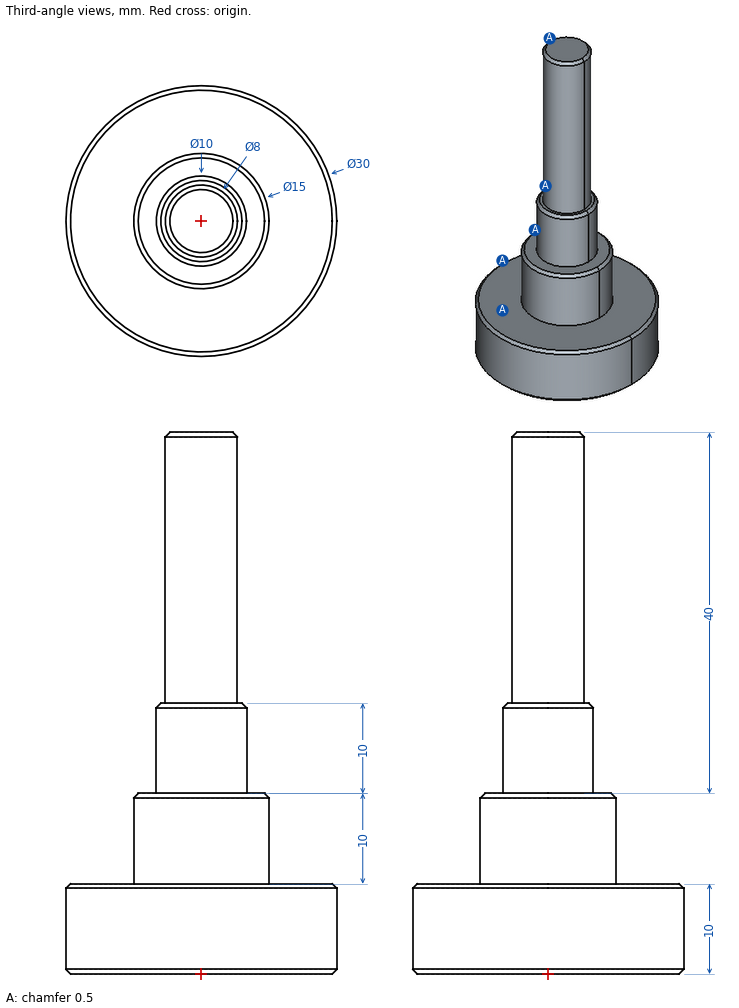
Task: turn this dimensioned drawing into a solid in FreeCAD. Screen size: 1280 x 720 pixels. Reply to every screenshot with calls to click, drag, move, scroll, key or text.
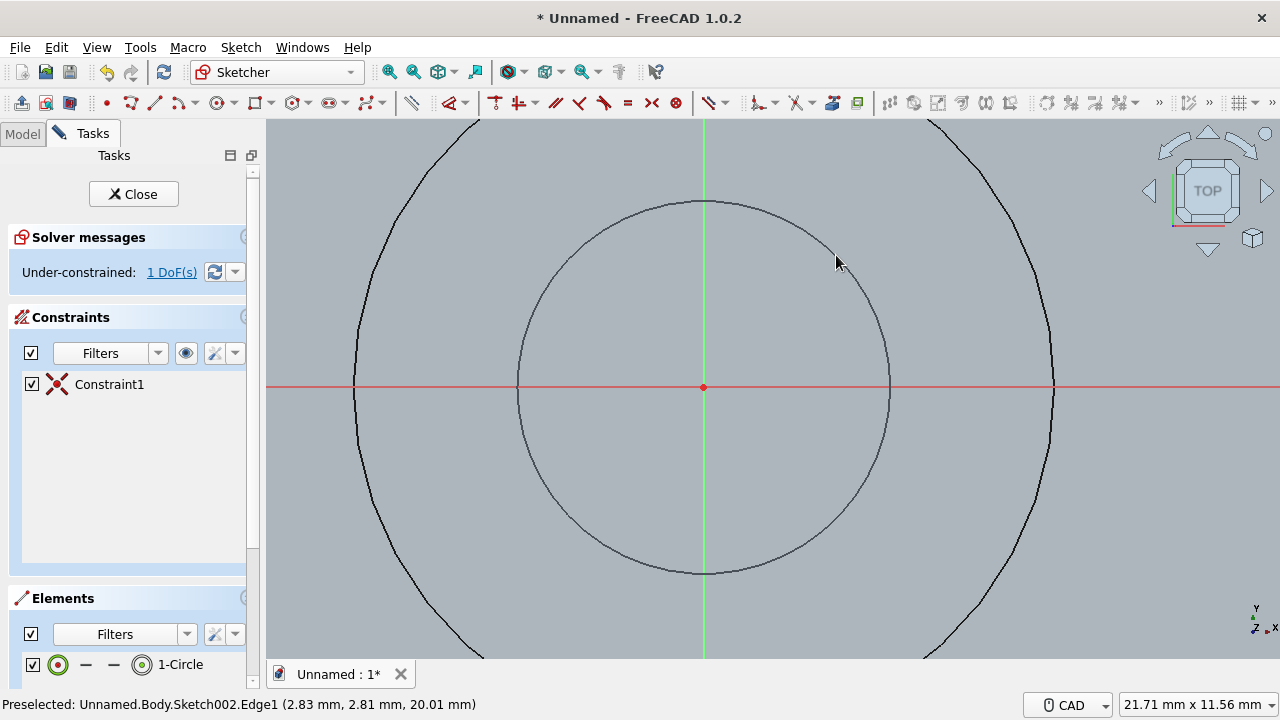
click(835, 255)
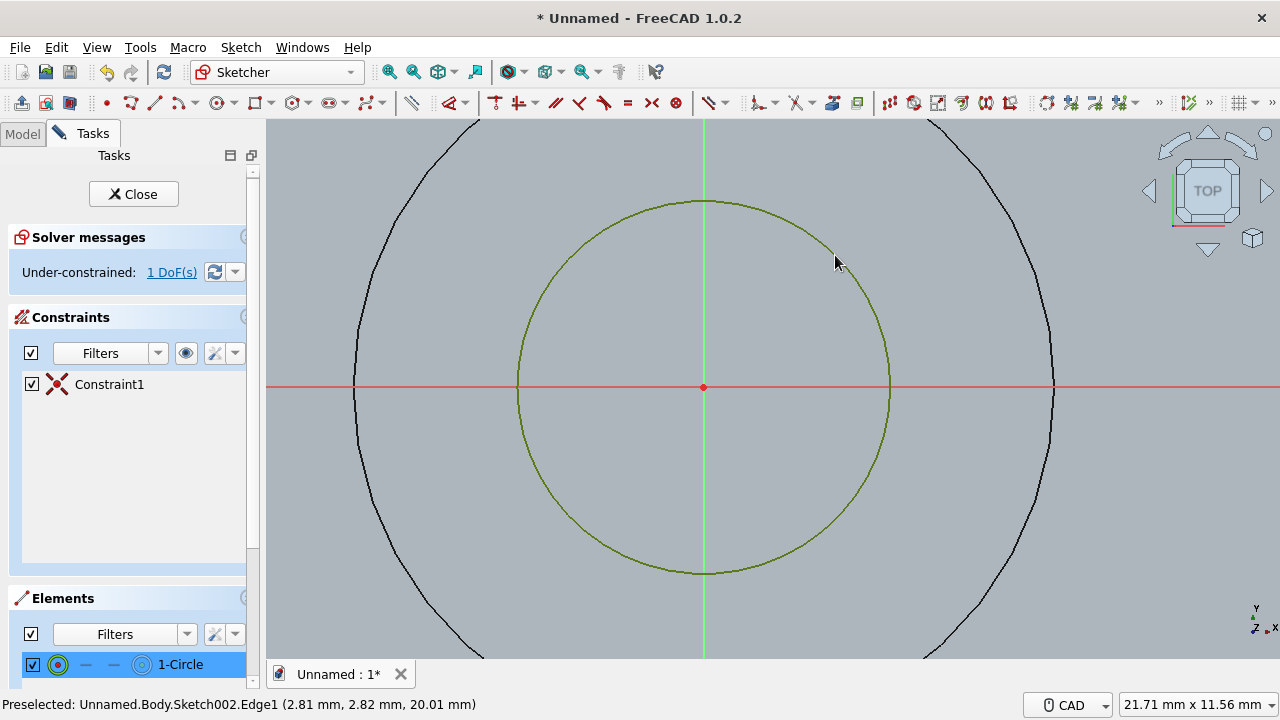
key(k)
key(o)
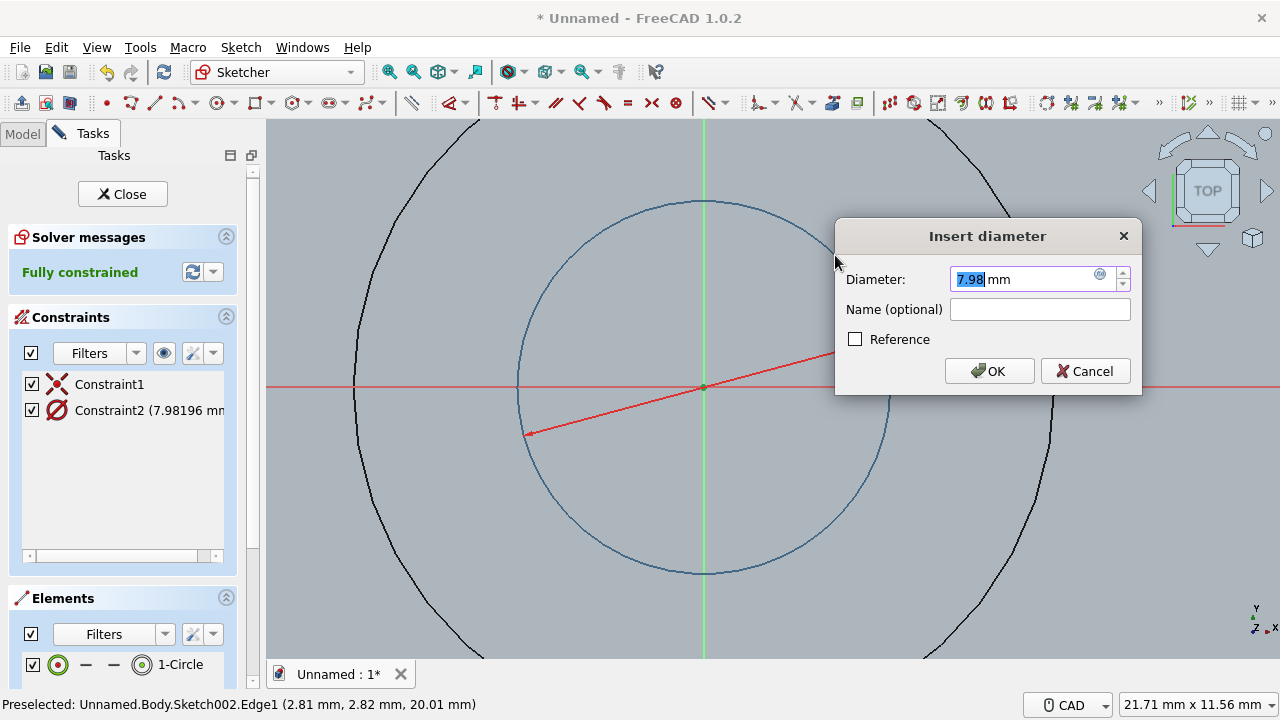
text(8)
key(Return)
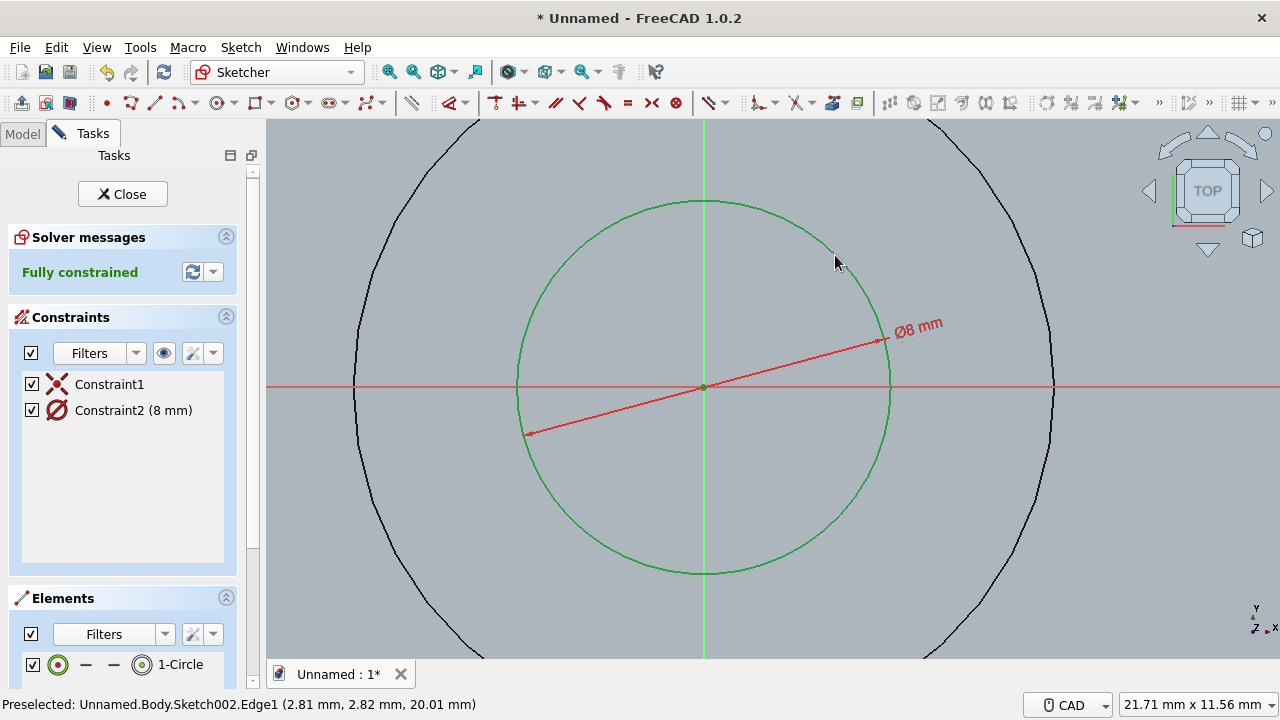
click(123, 194)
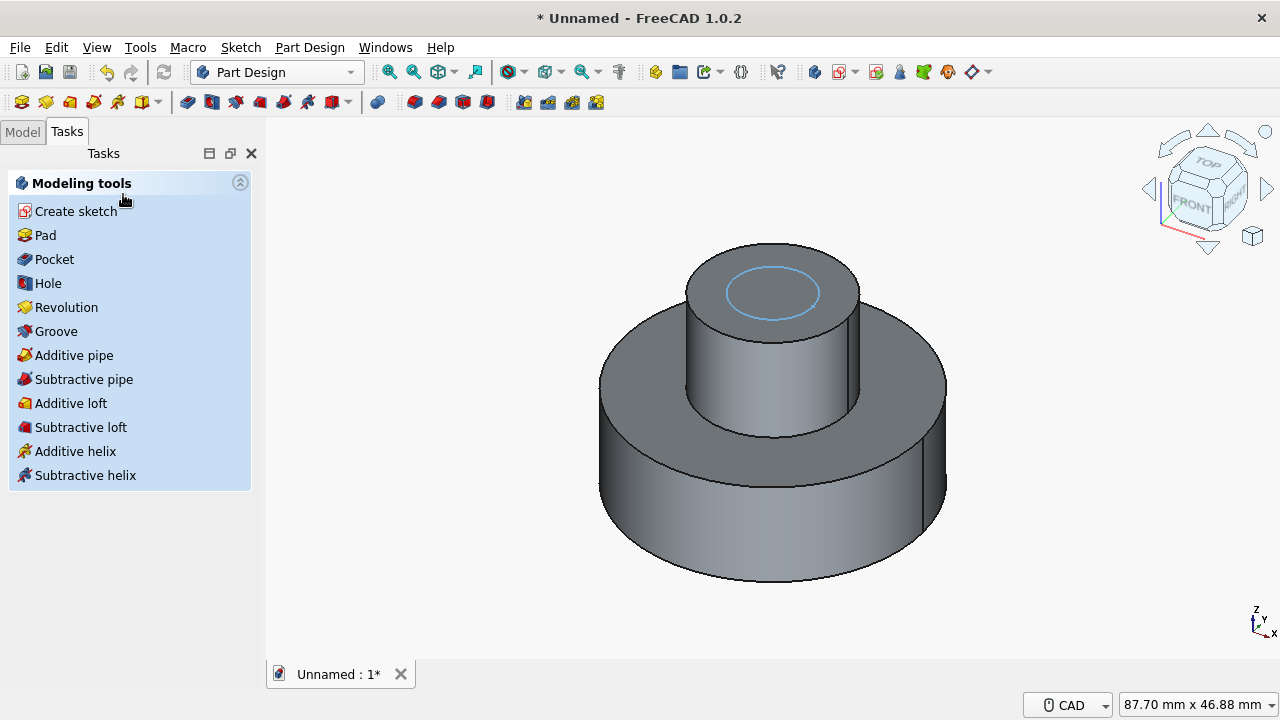
click(22, 102)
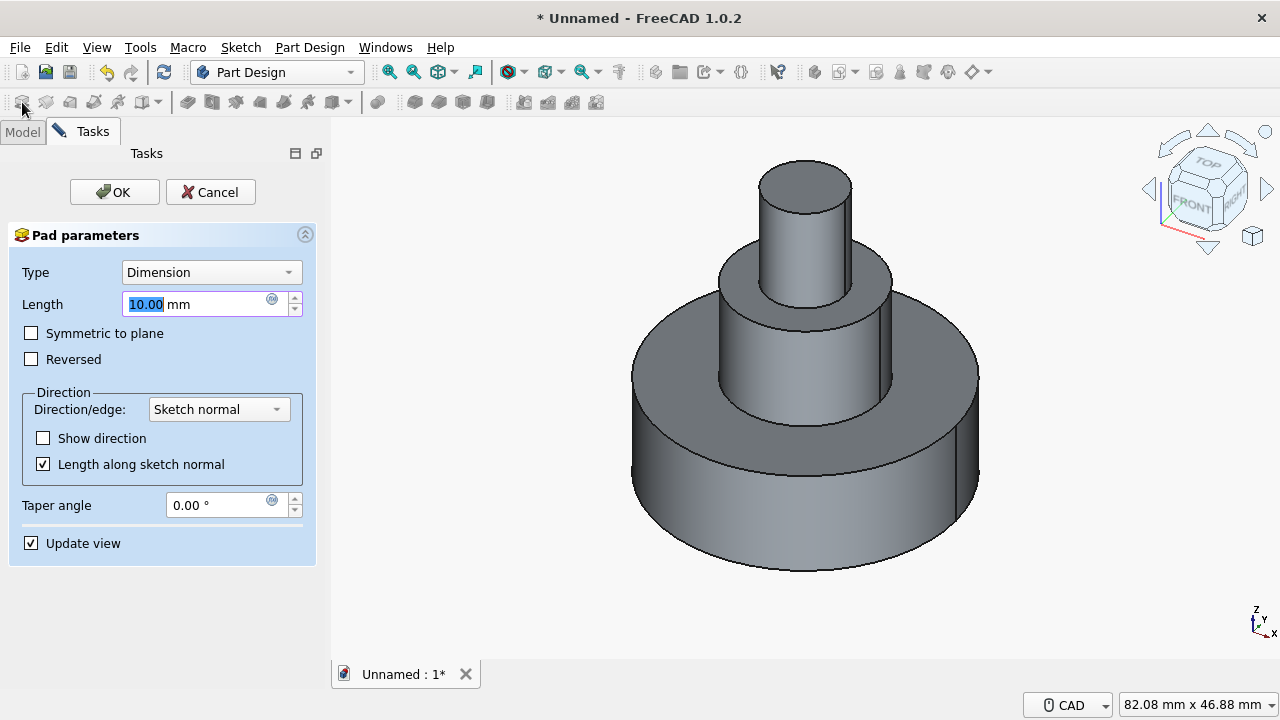
text(40)
key(Tab)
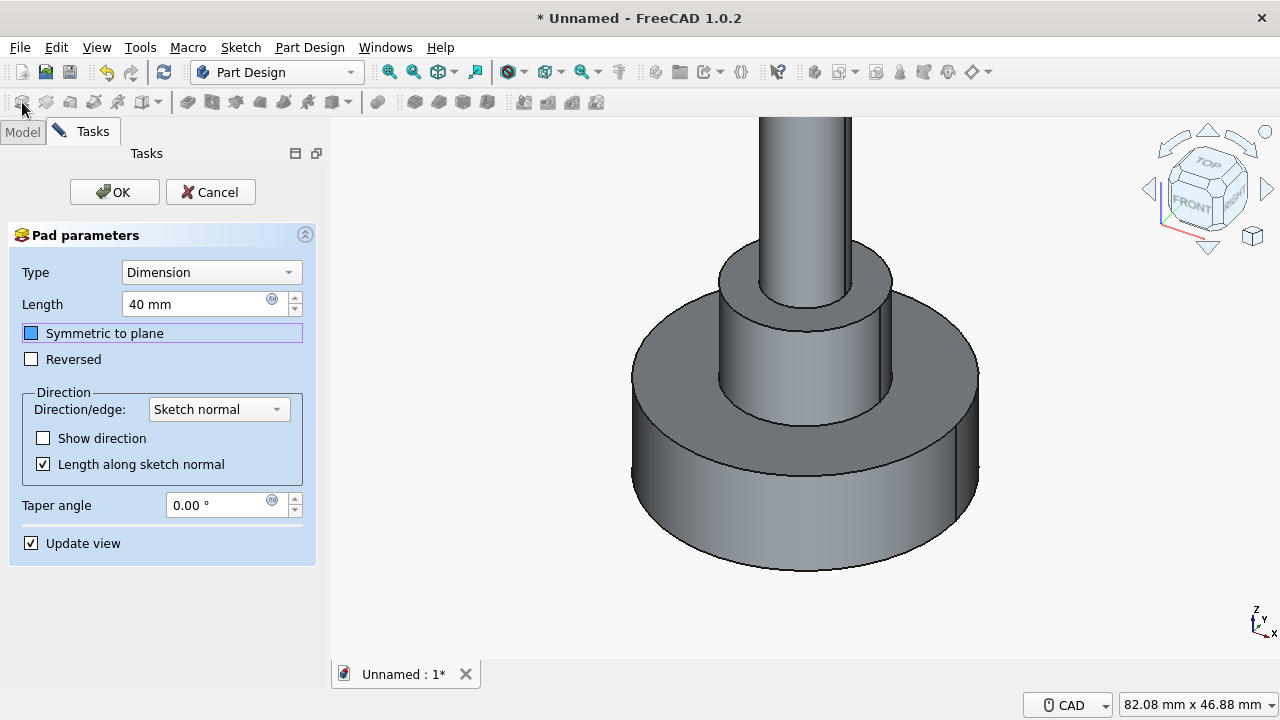
click(115, 192)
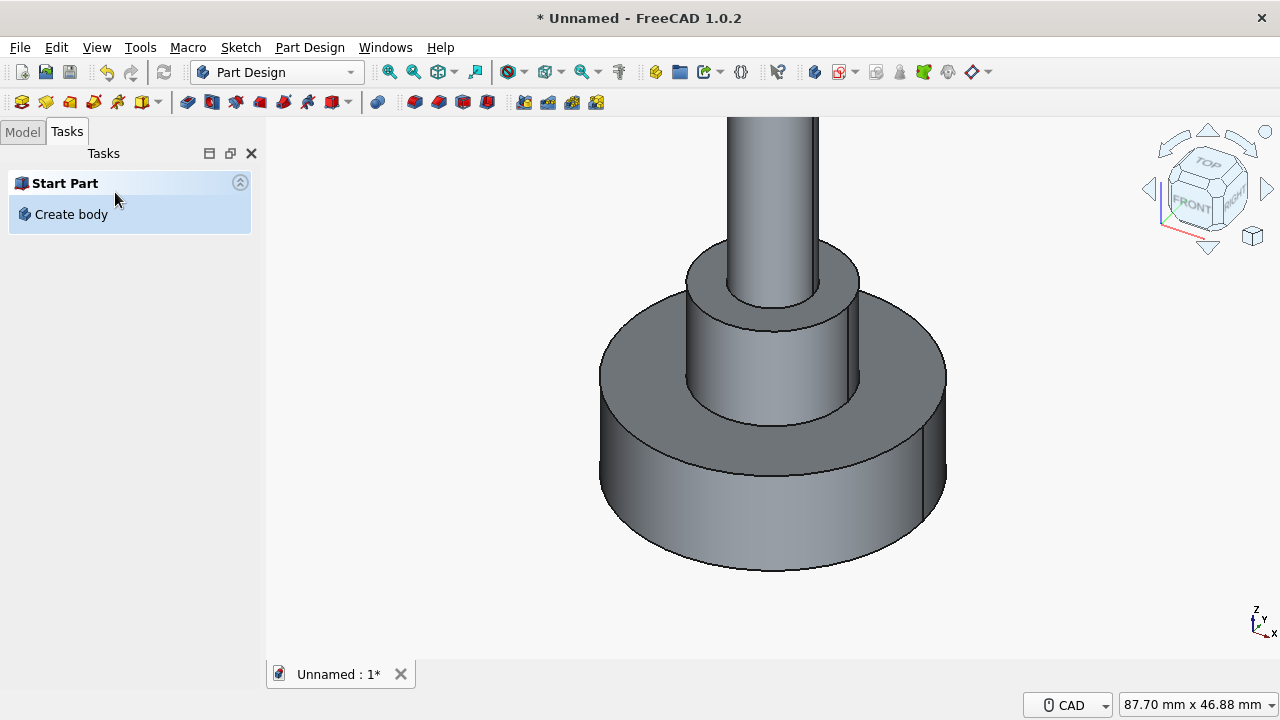
click(390, 72)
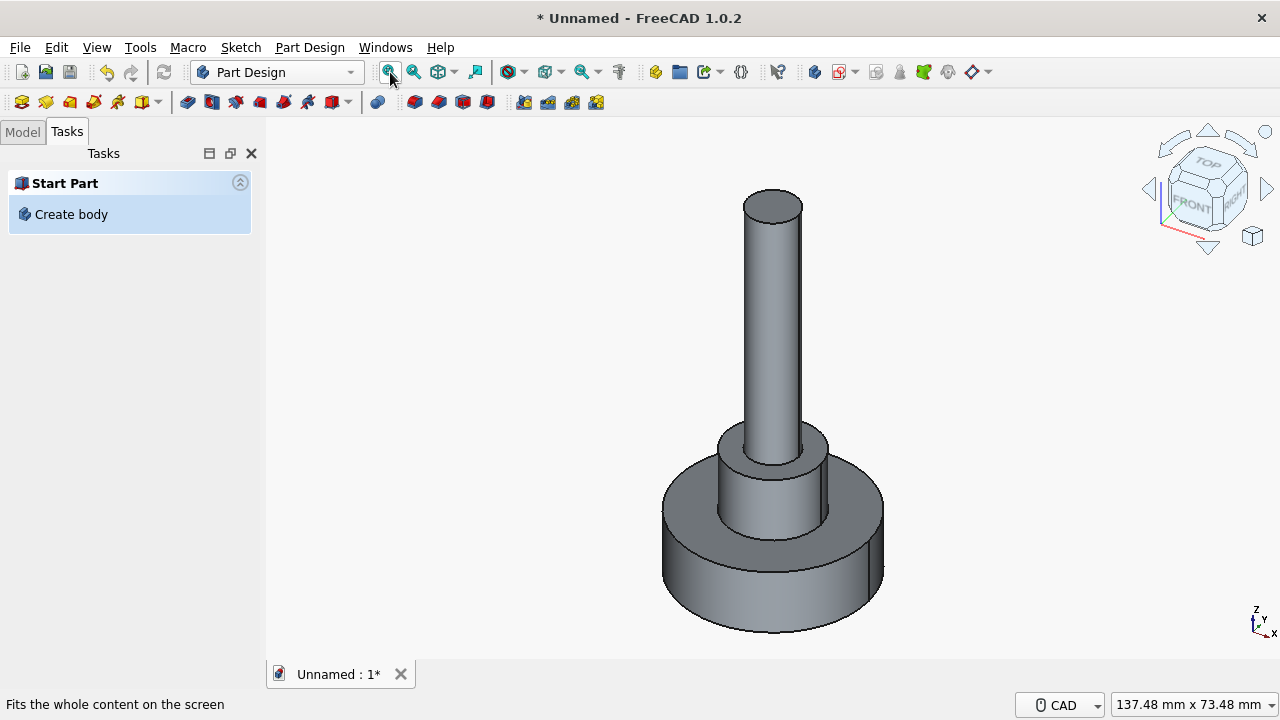
click(730, 454)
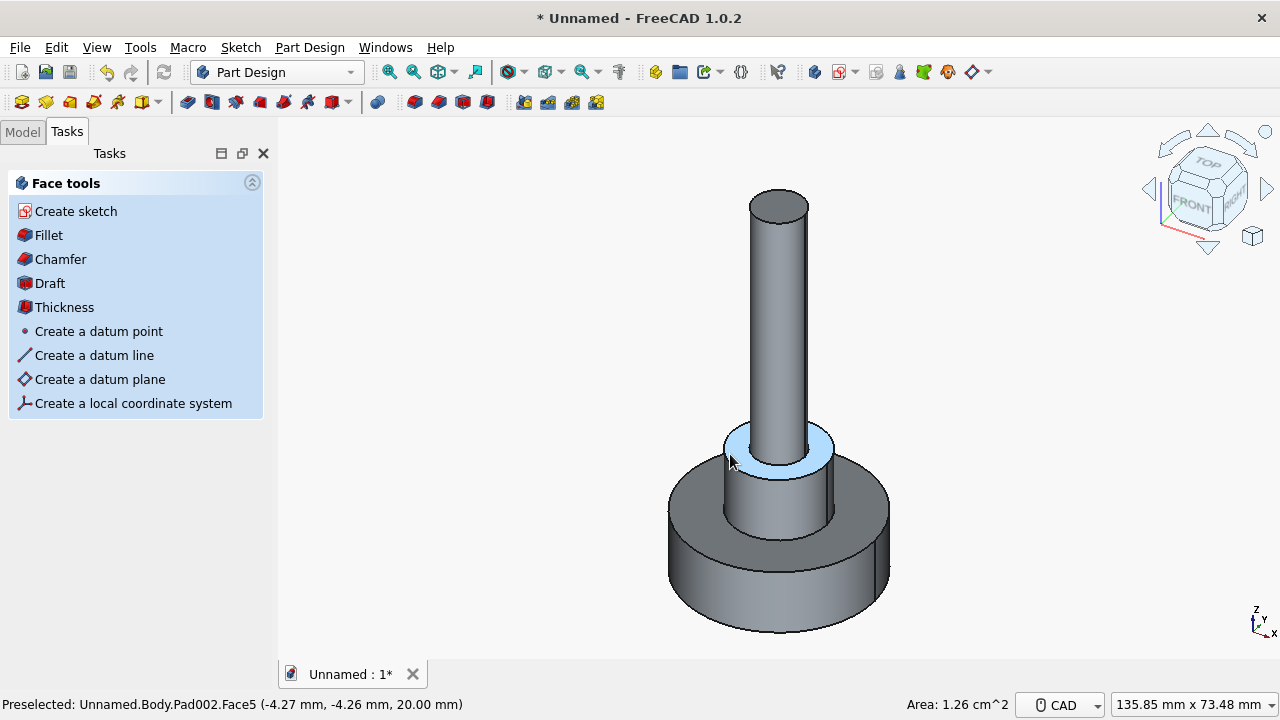
click(840, 72)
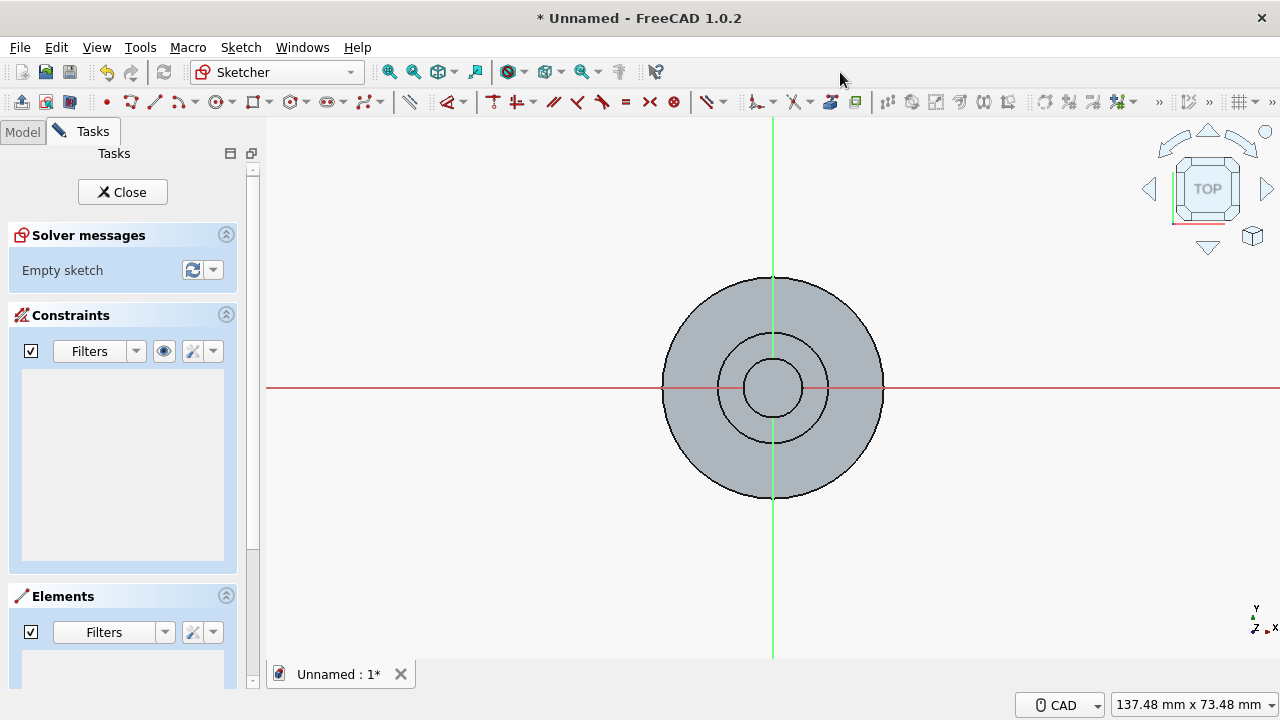
scroll(790, 388, up, 8)